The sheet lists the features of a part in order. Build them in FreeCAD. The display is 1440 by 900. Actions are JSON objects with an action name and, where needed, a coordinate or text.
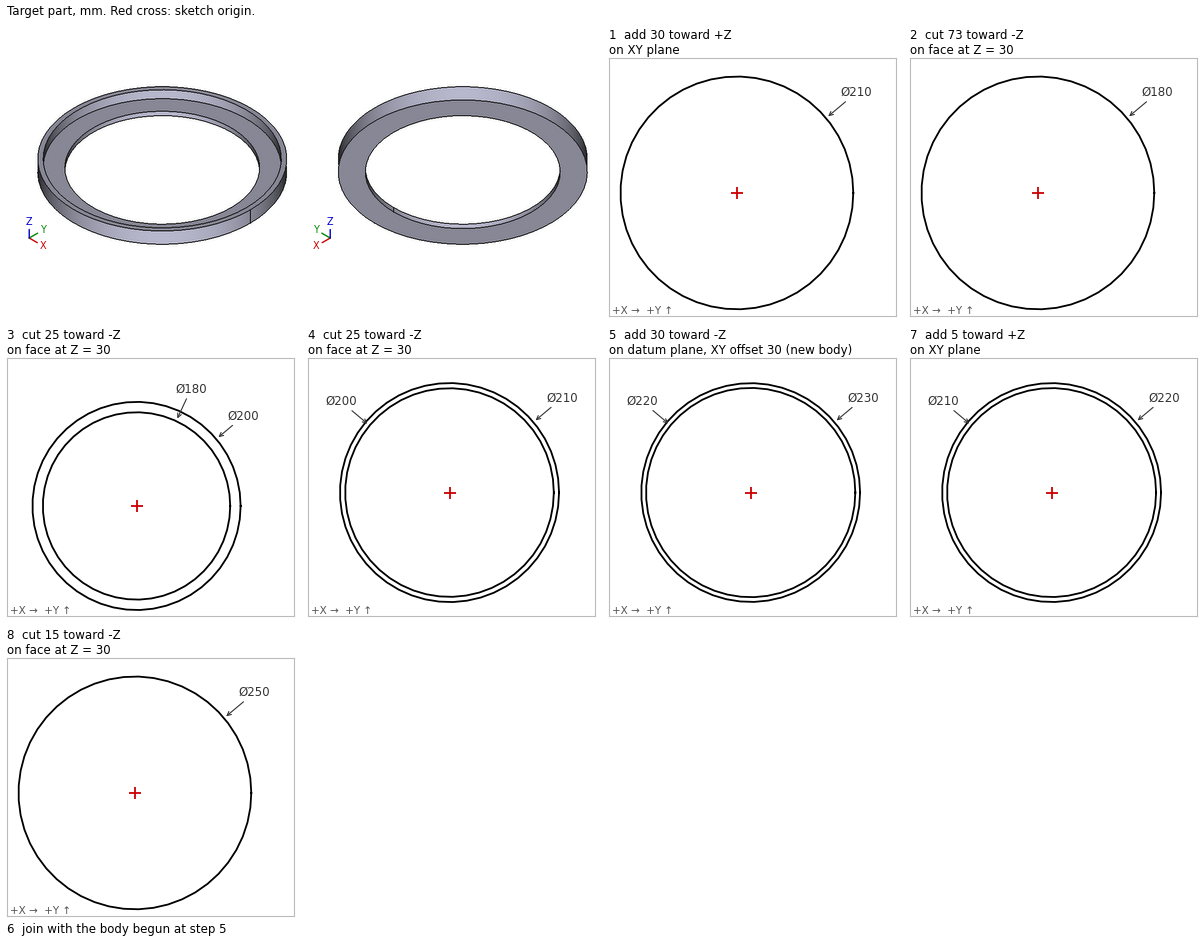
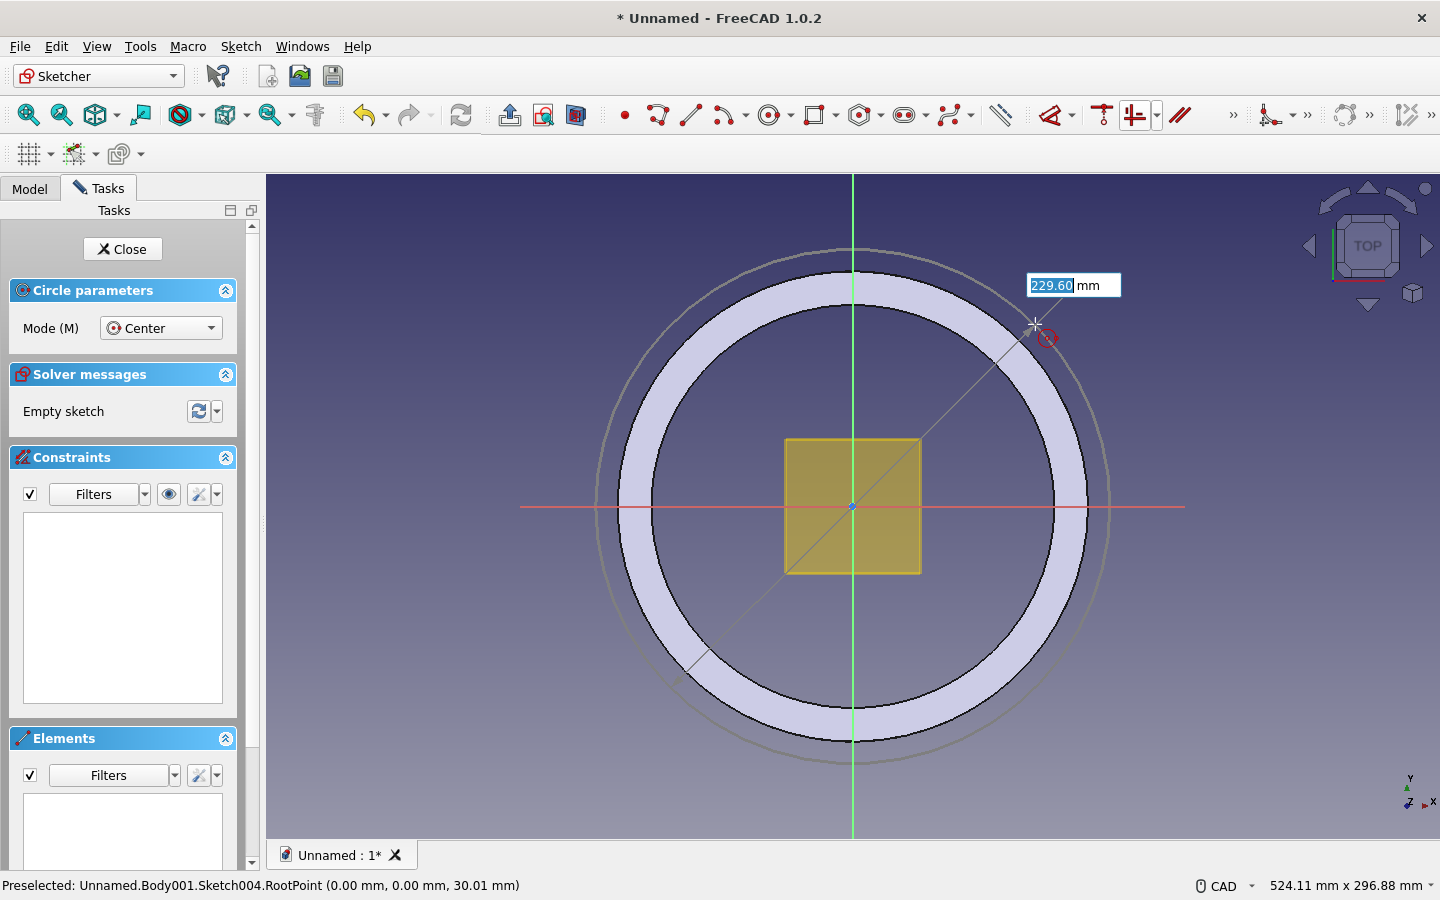
{"action": "type", "text": "230"}
{"action": "key", "text": "Return"}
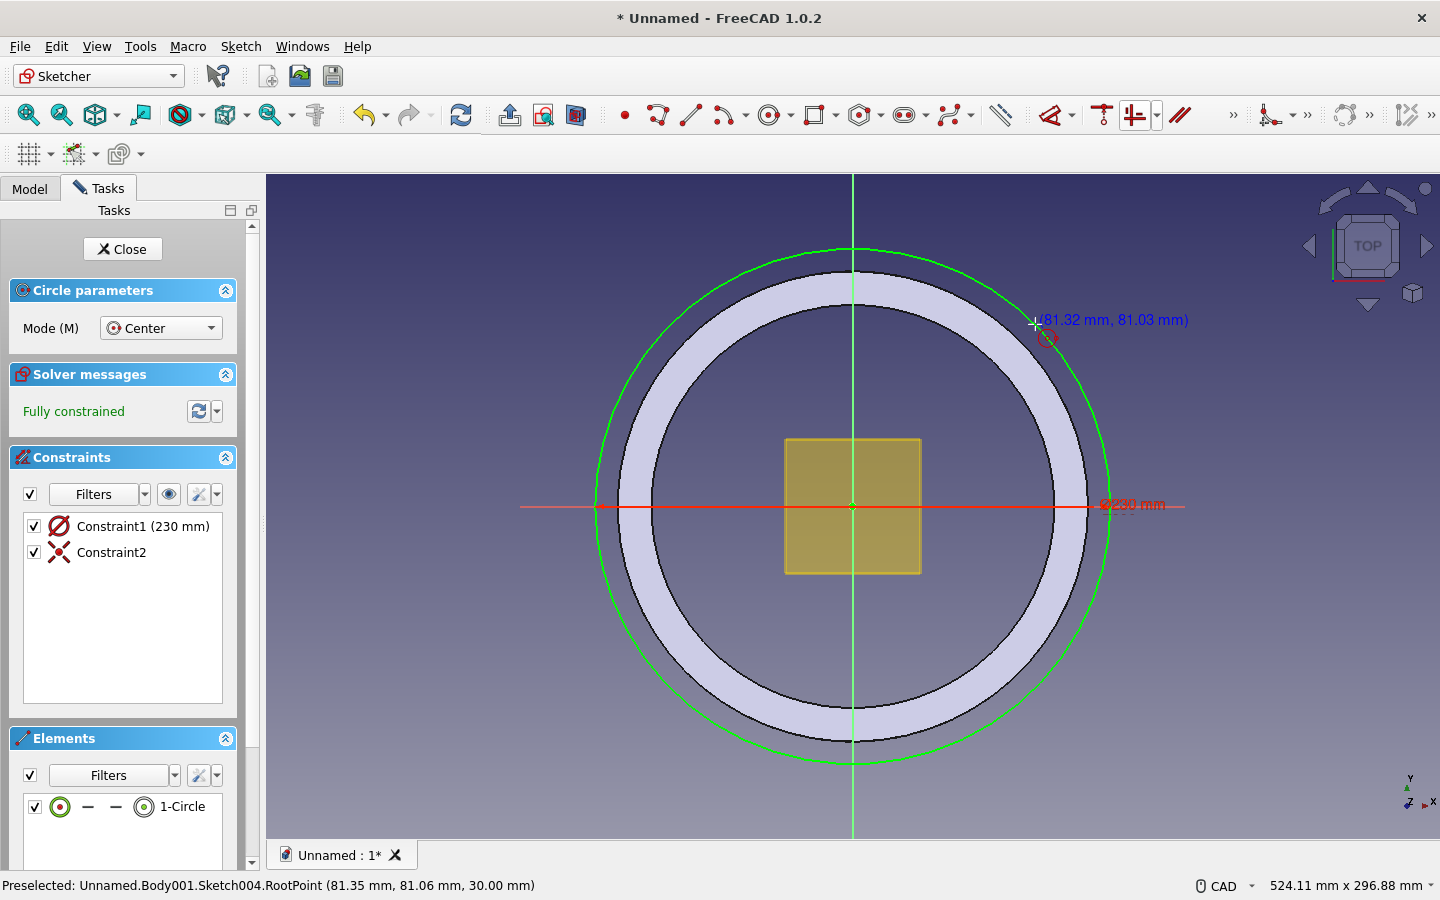
{"action": "left_click", "coordinate": [853, 506]}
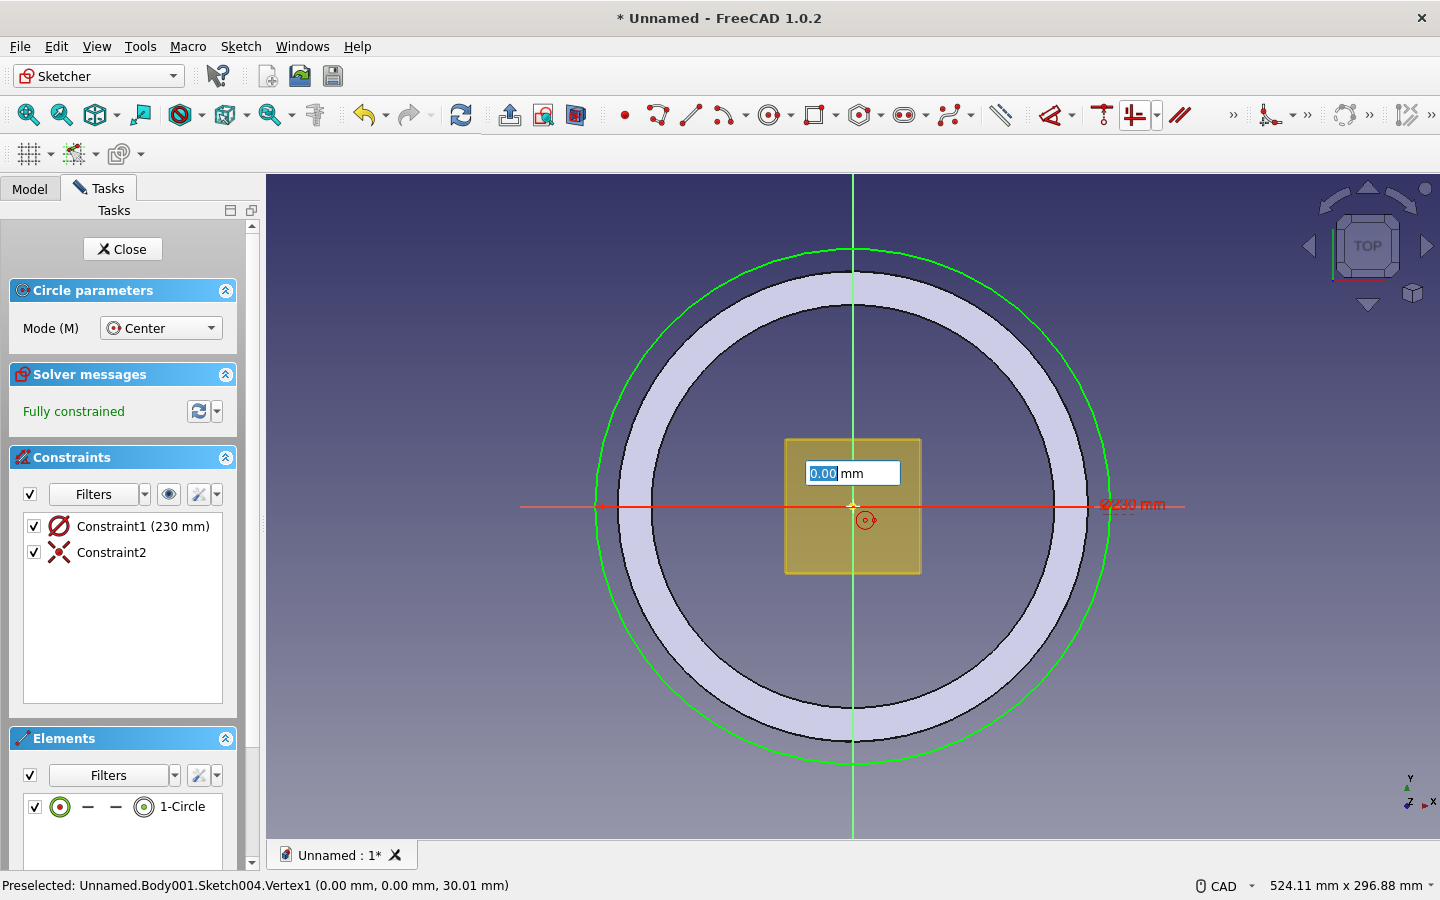
{"action": "scroll", "coordinate": [1027, 332], "scroll_direction": "up", "scroll_amount": 2}
{"action": "mouse_move", "coordinate": [1027, 332]}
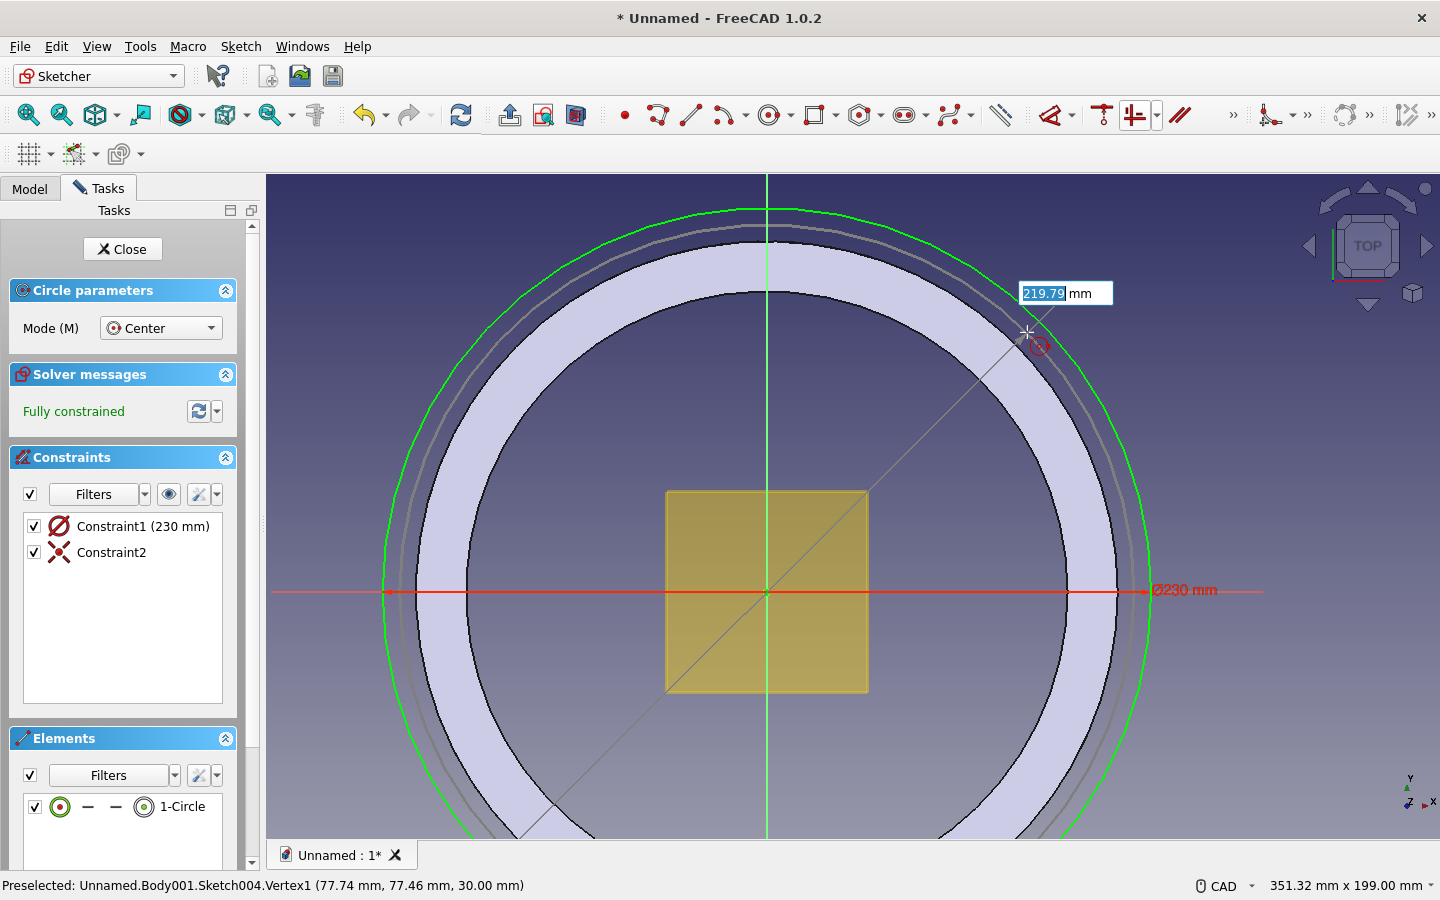
{"action": "type", "text": "220"}
{"action": "key", "text": "Return"}
{"action": "key", "text": "Escape"}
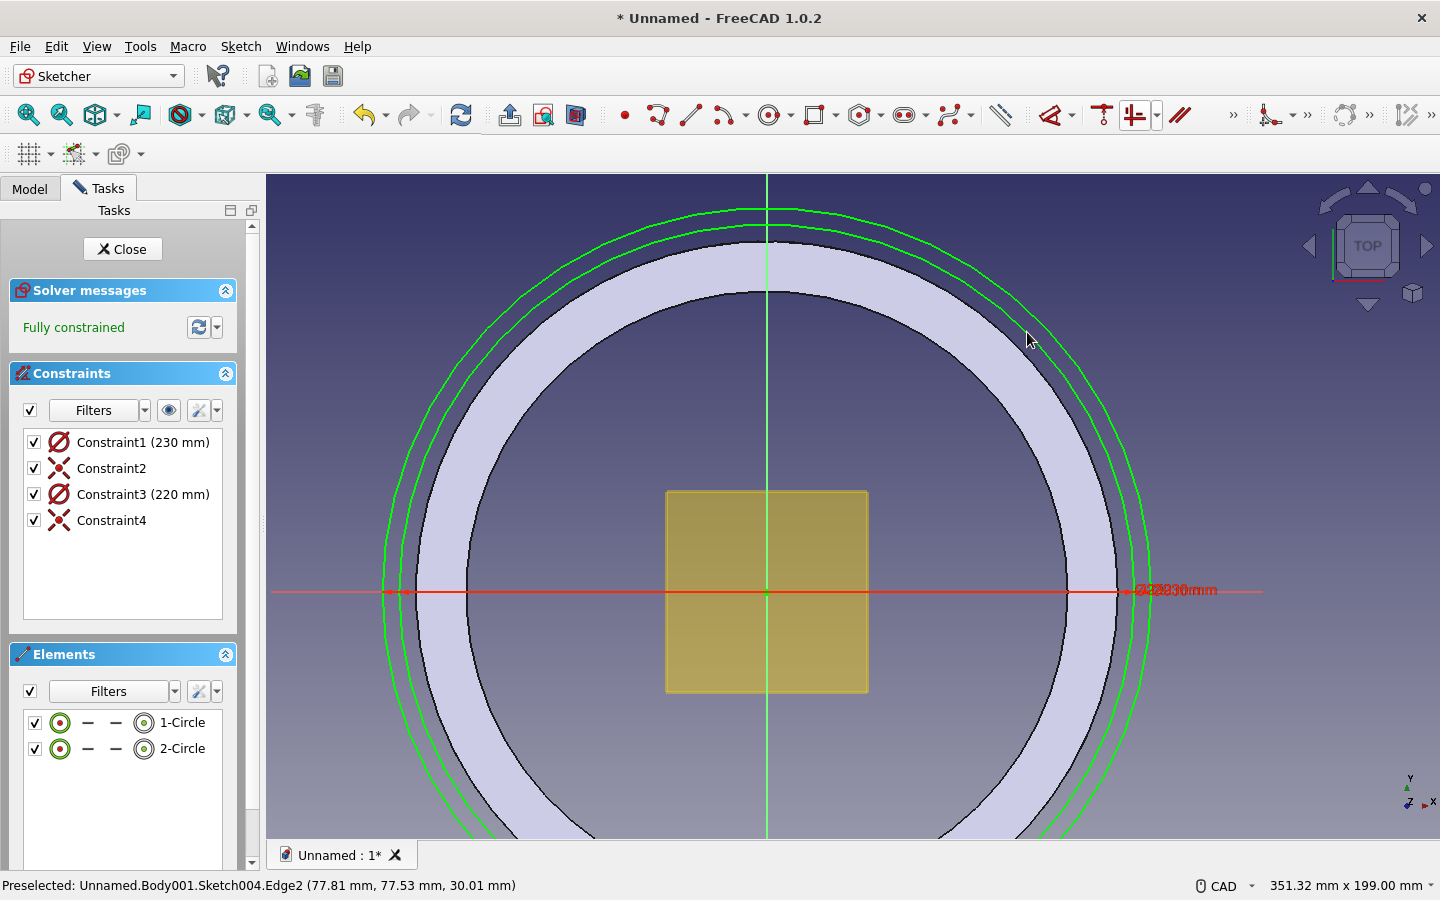
{"action": "left_click", "coordinate": [123, 249]}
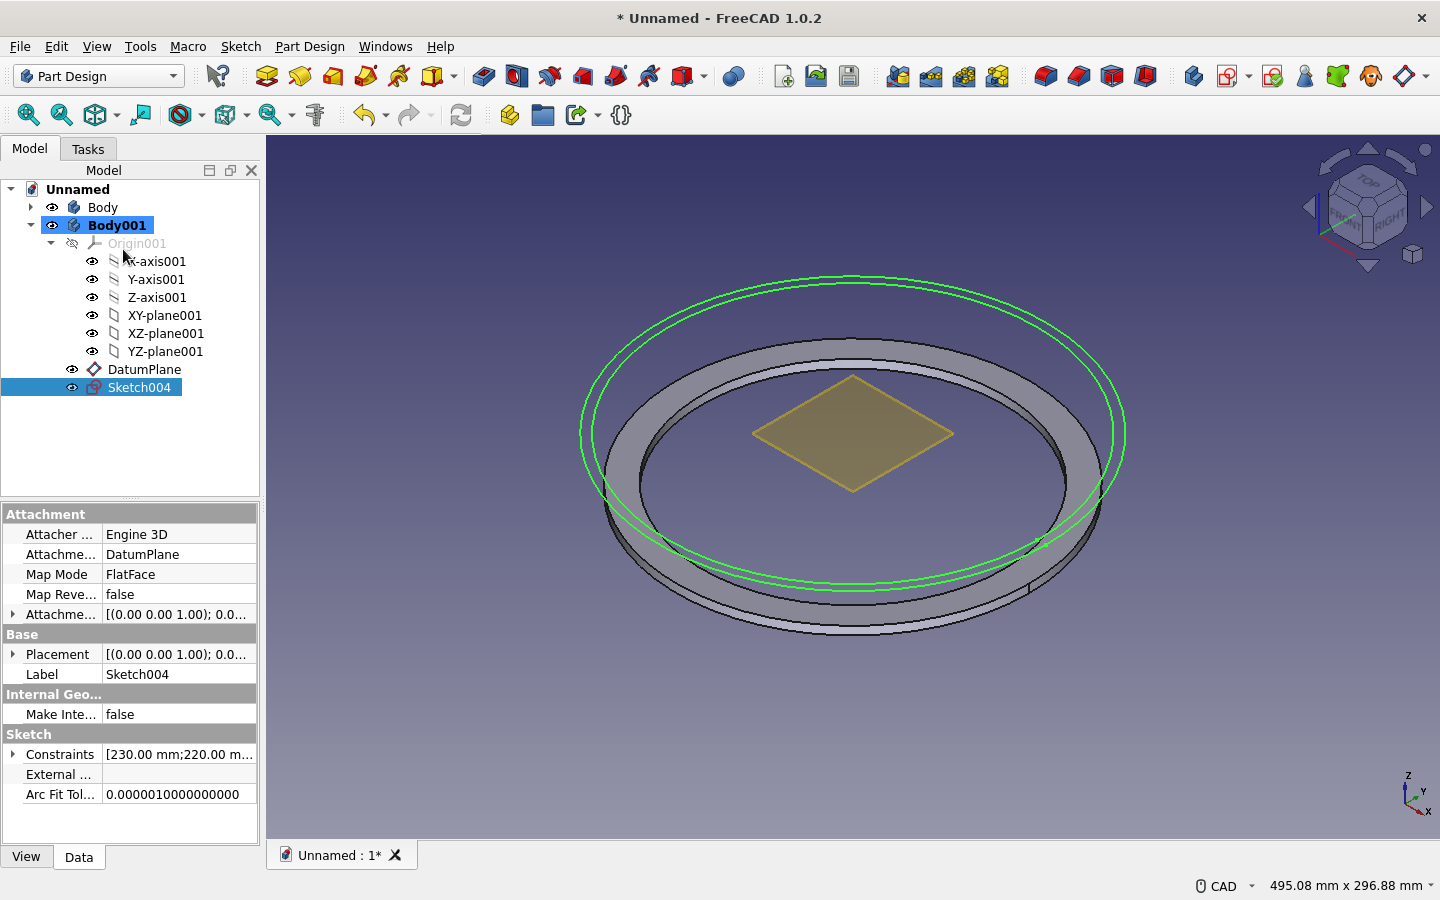
{"action": "left_click", "coordinate": [267, 76]}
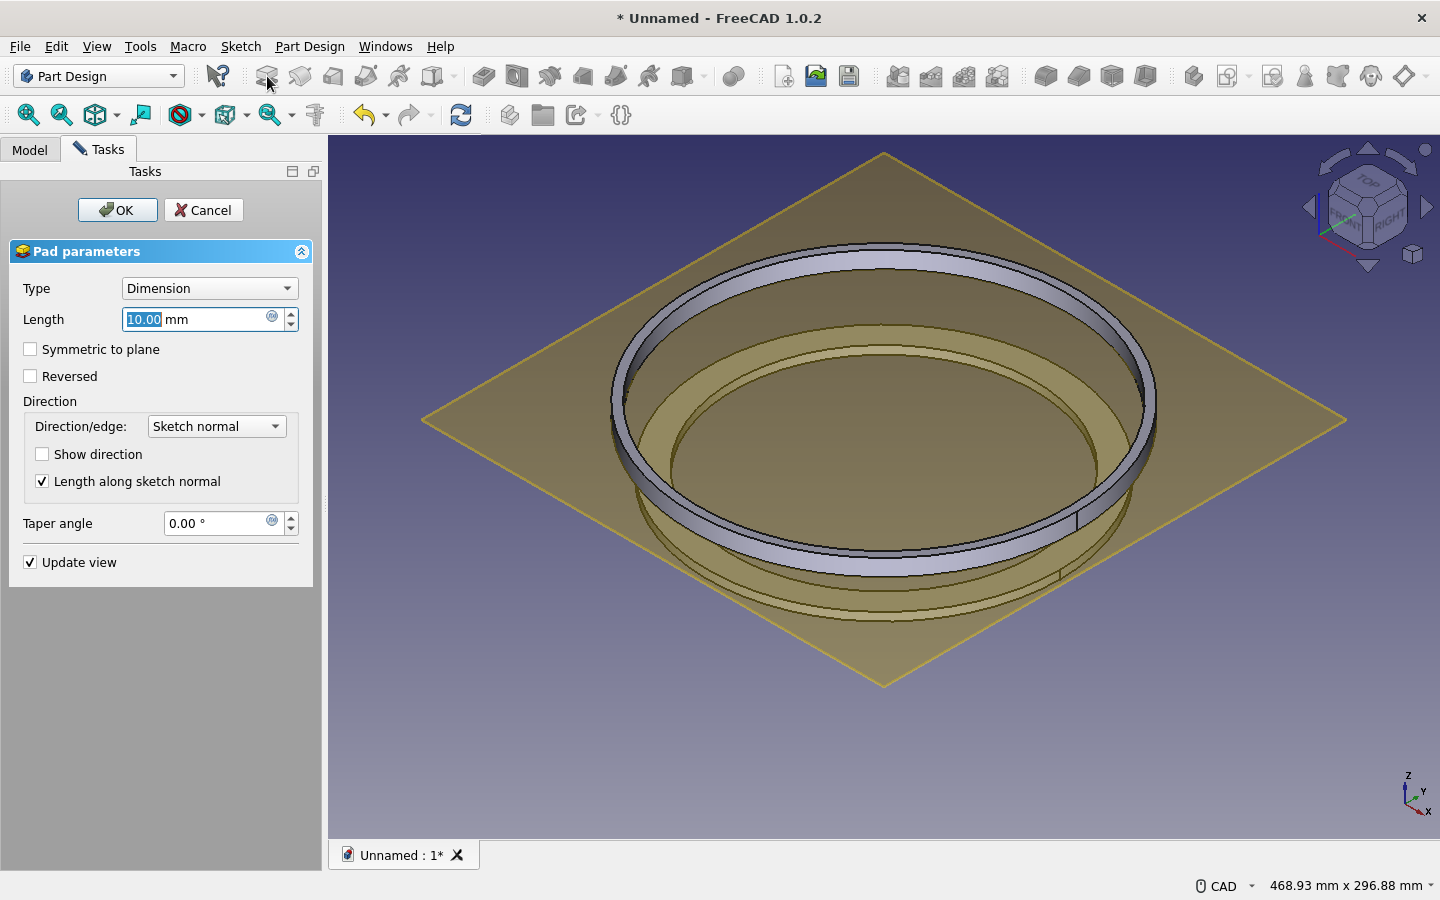
{"action": "type", "text": "30"}
{"action": "key", "text": "Tab"}